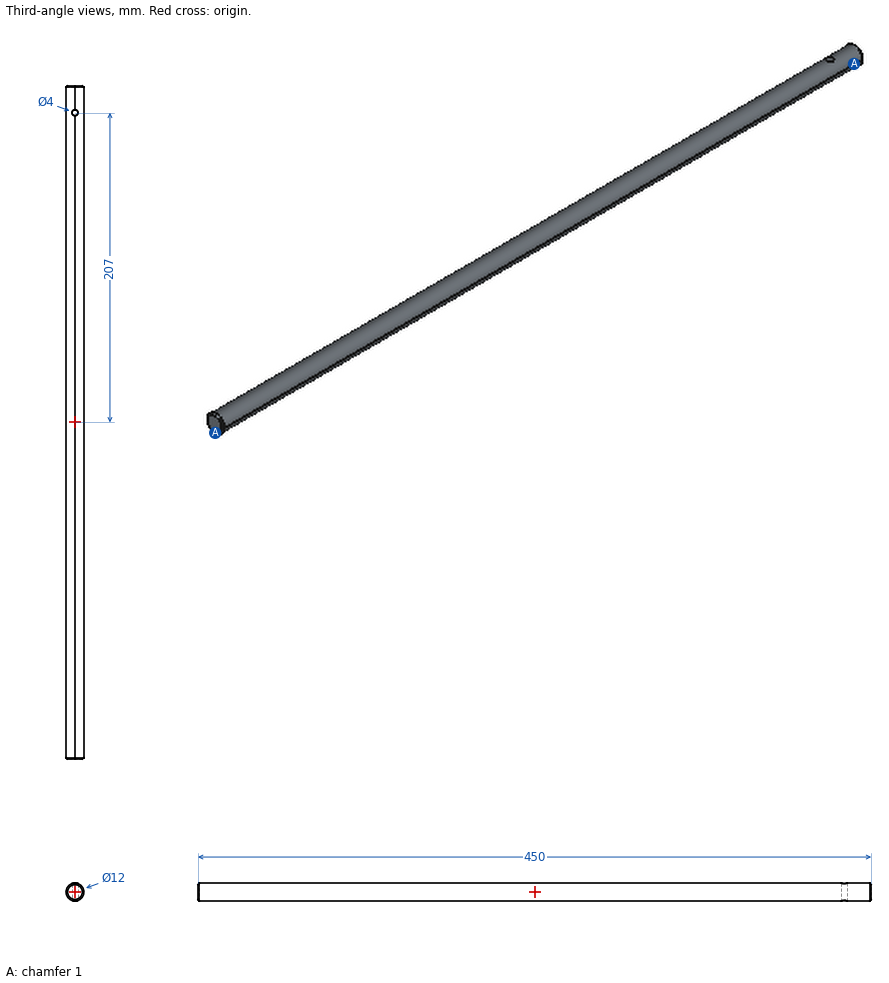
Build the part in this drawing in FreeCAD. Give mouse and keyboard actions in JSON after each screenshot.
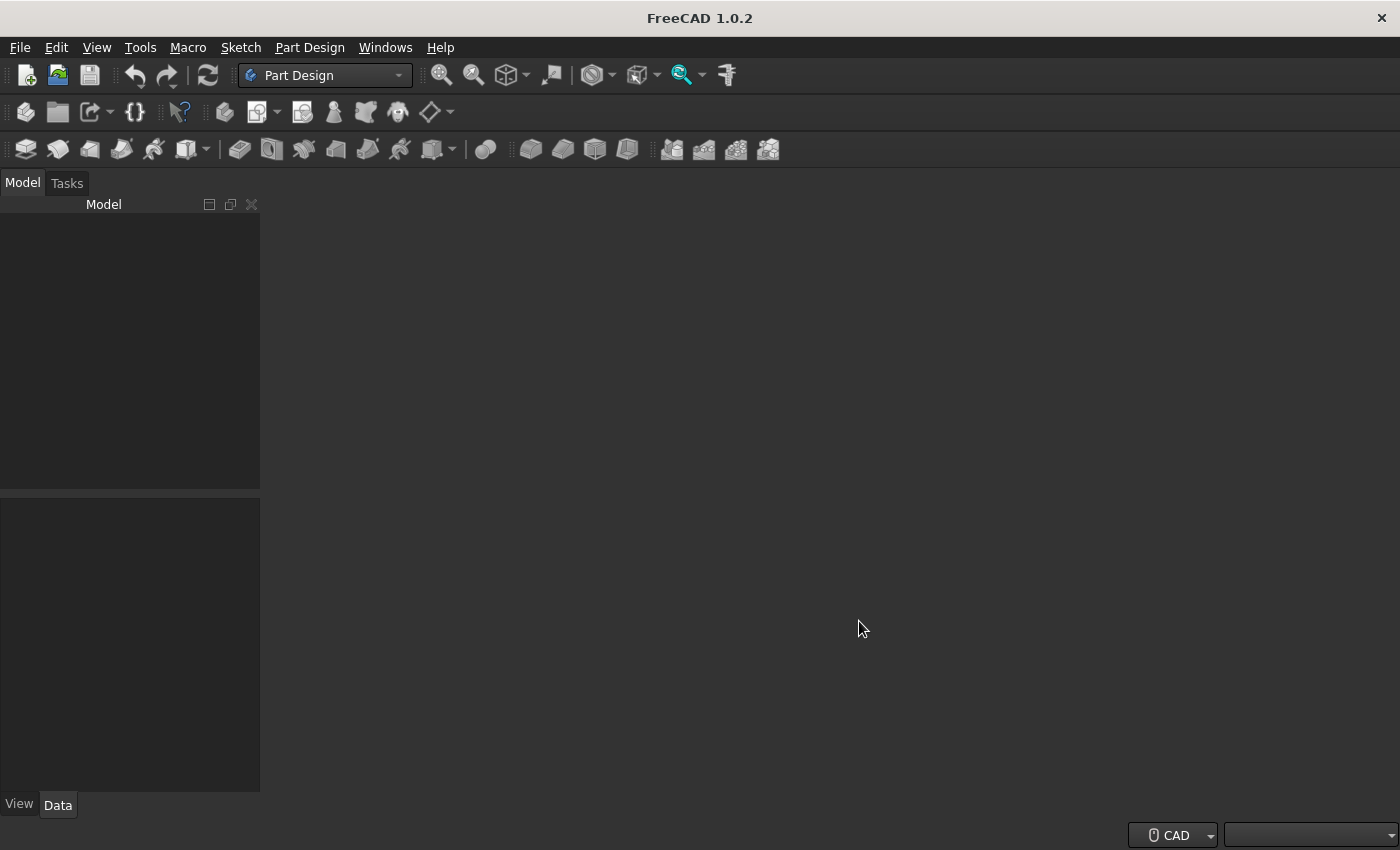
{"action": "key", "text": "ctrl+n"}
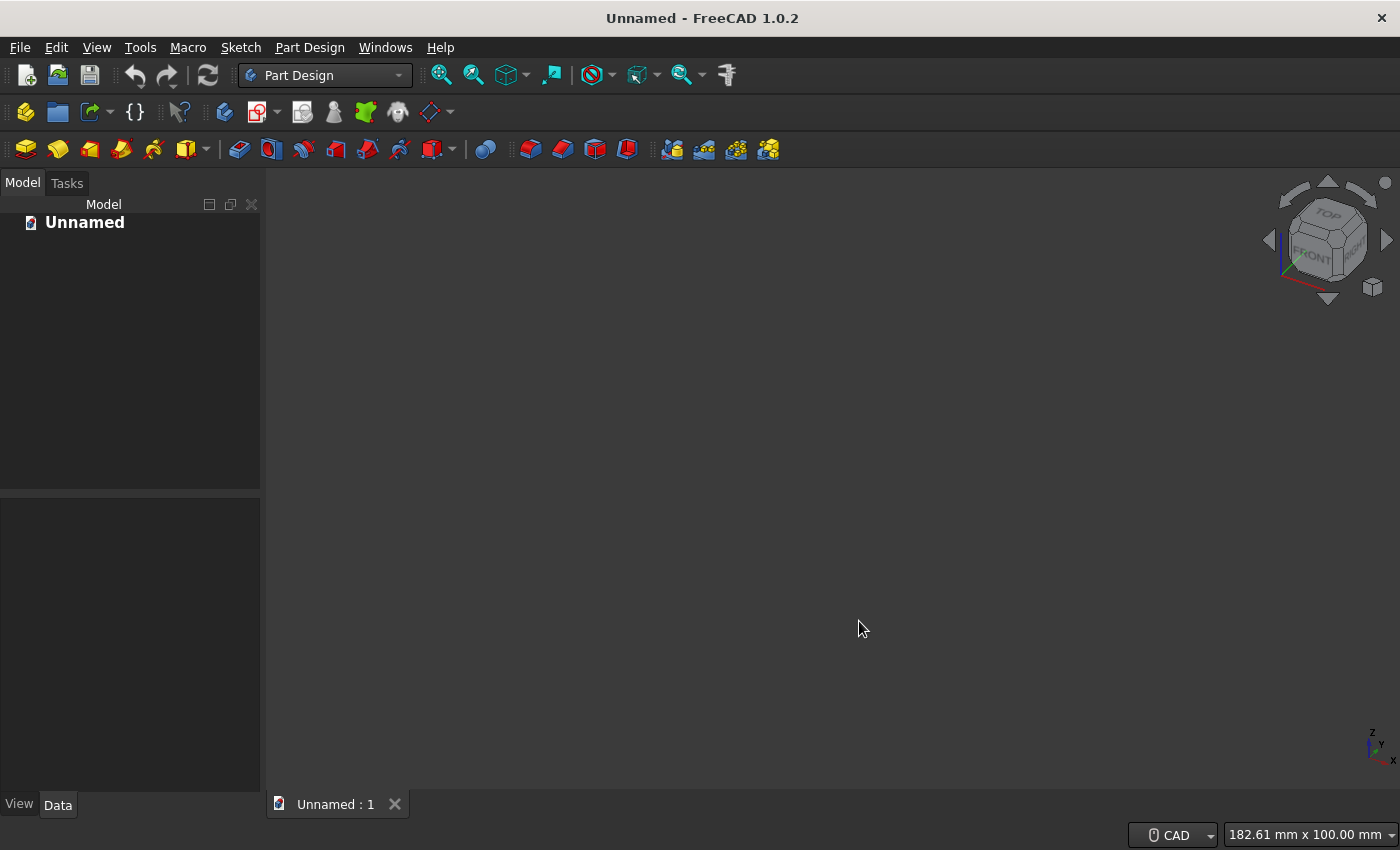
{"action": "left_click", "coordinate": [258, 112]}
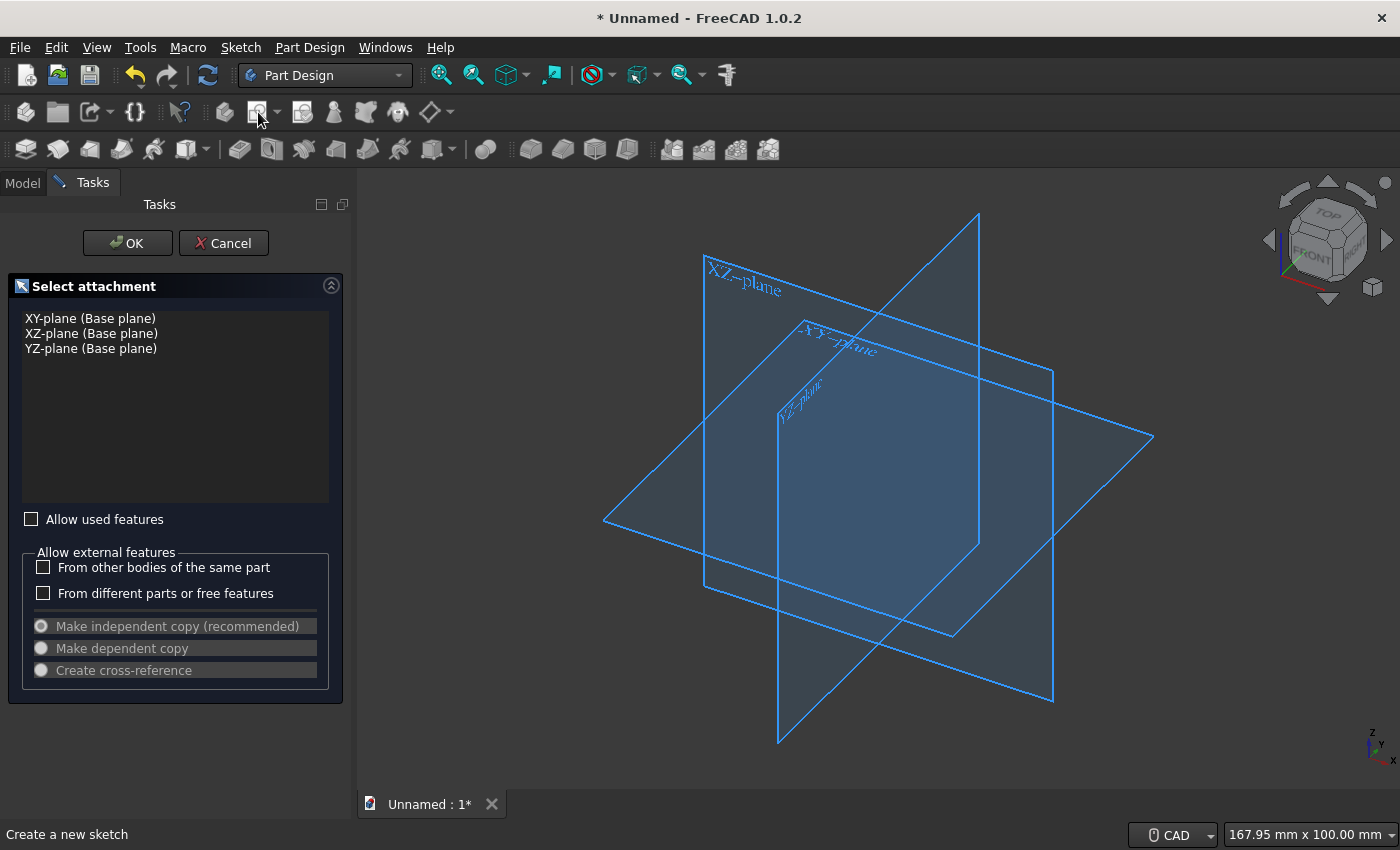
{"action": "left_click", "coordinate": [82, 334]}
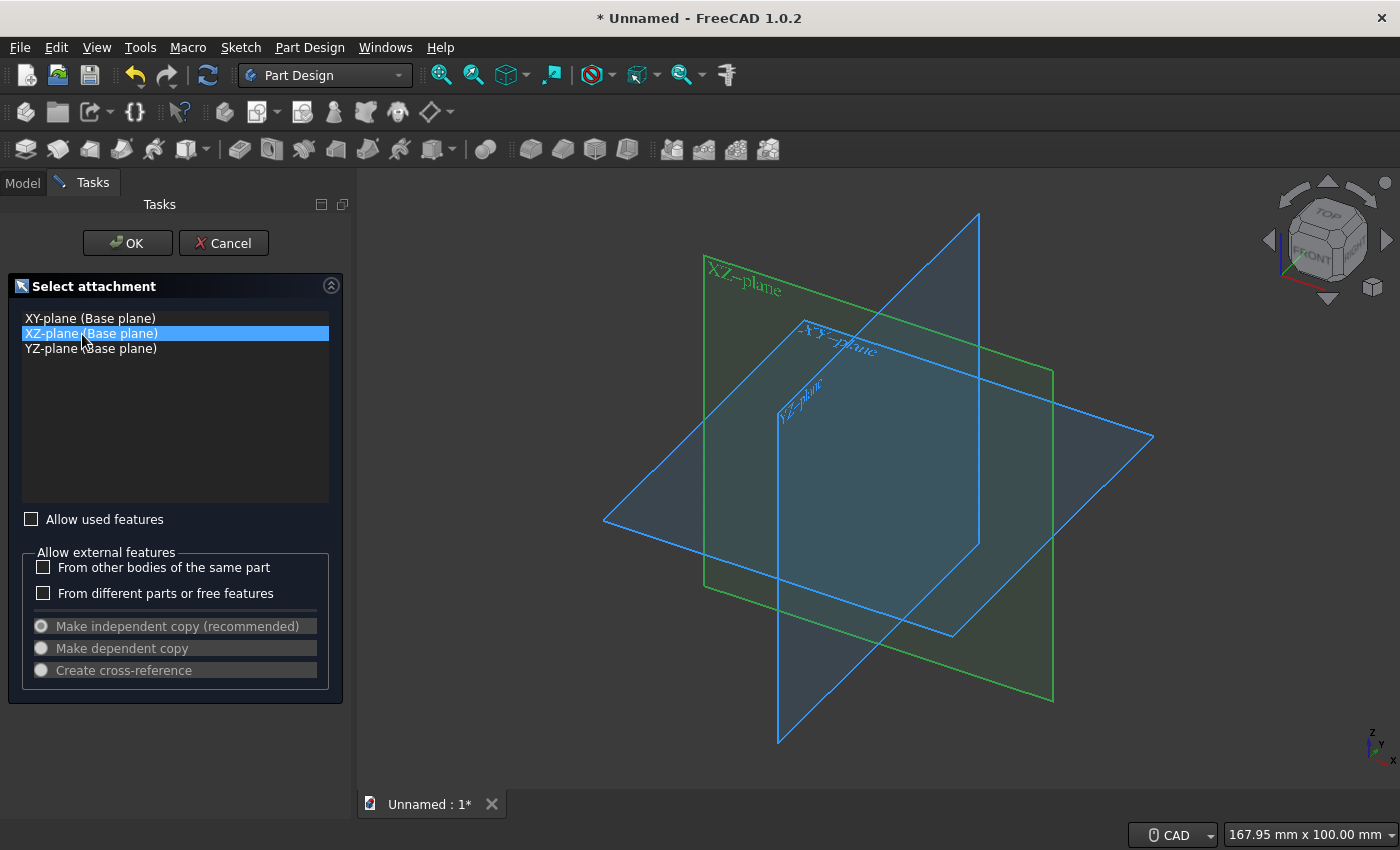
{"action": "left_click", "coordinate": [128, 243]}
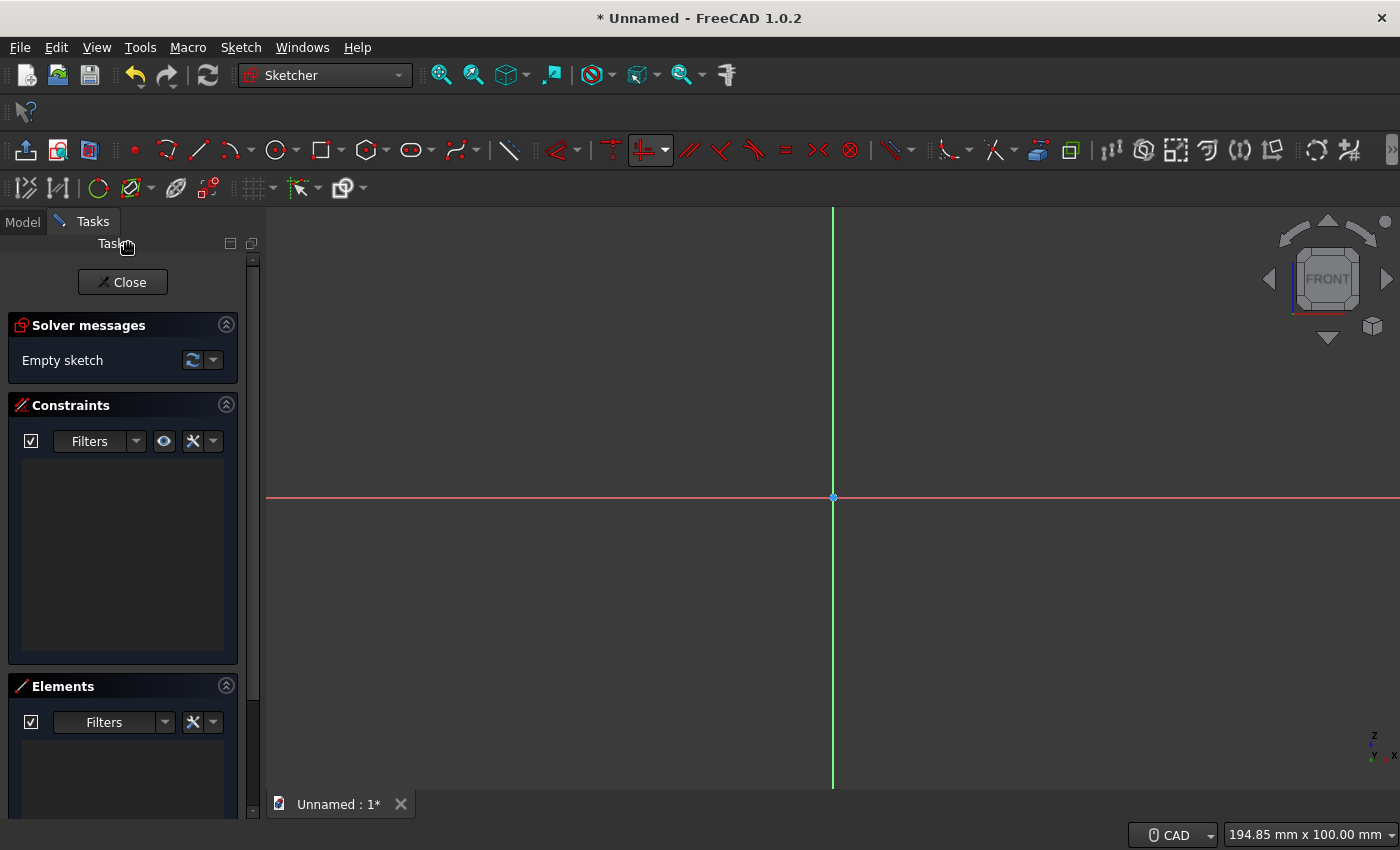
{"action": "scroll", "coordinate": [850, 498], "scroll_direction": "up", "scroll_amount": 8}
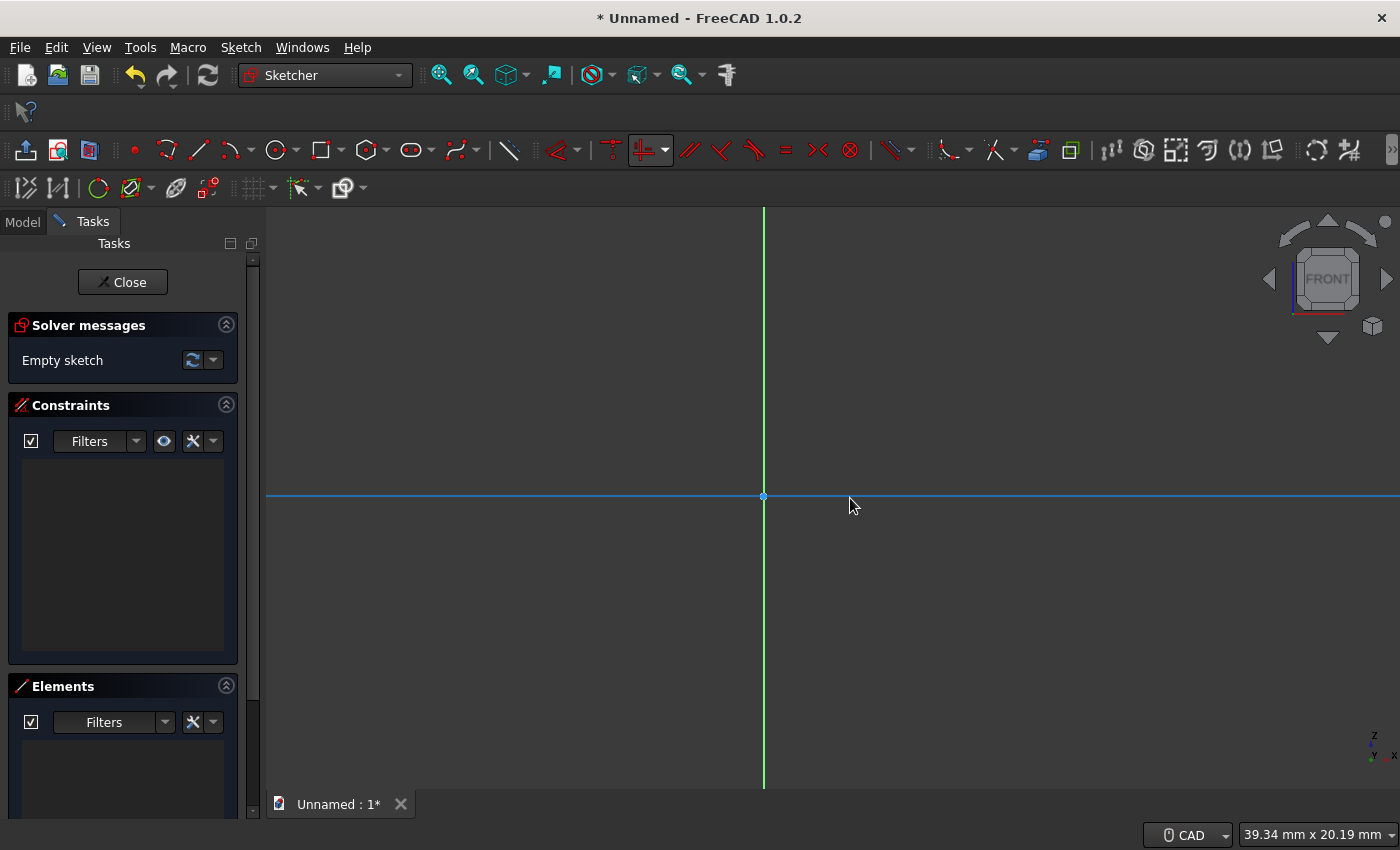
{"action": "key", "text": "g c"}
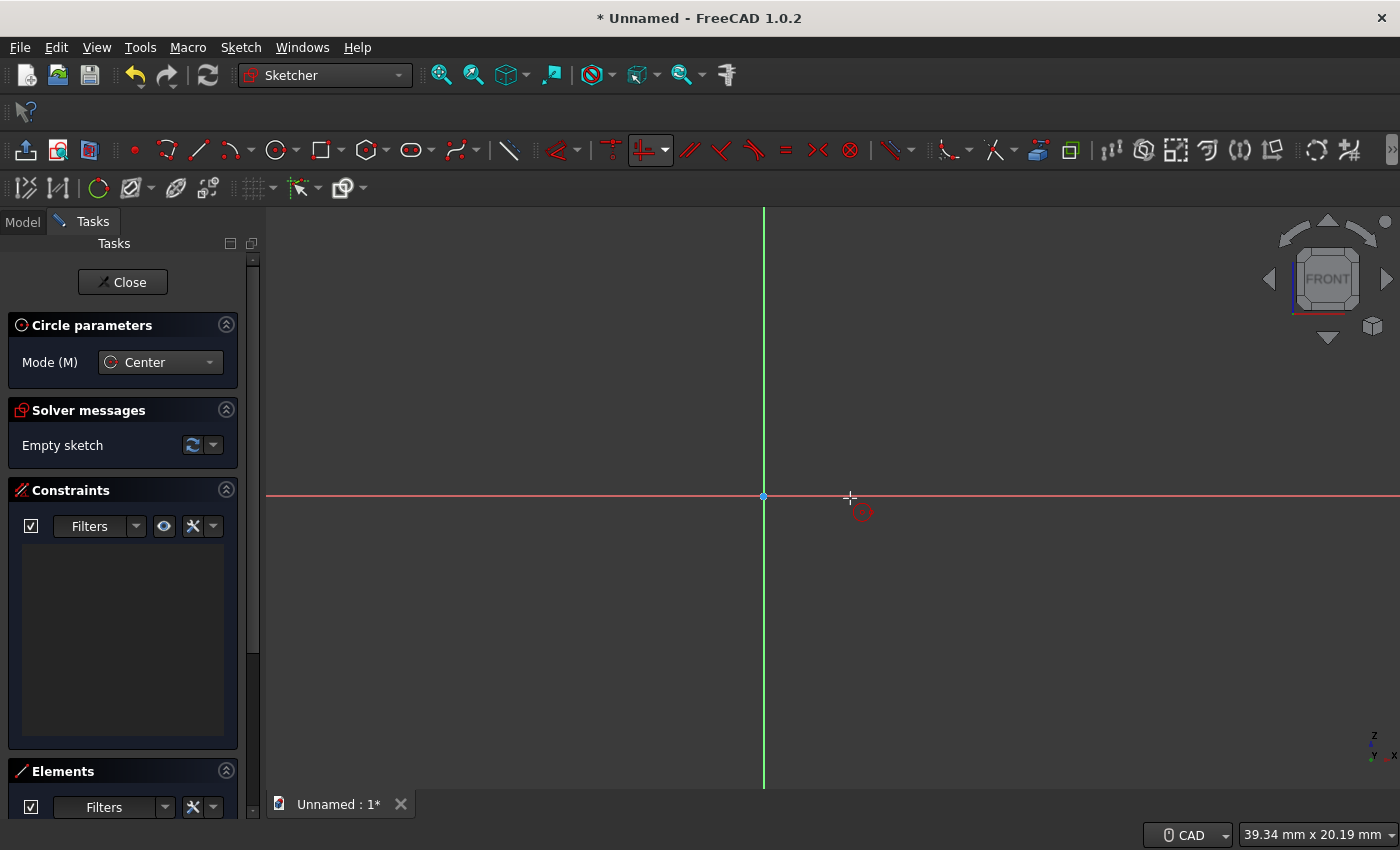
{"action": "left_click", "coordinate": [764, 496]}
{"action": "left_click", "coordinate": [886, 374]}
{"action": "key", "text": "Escape"}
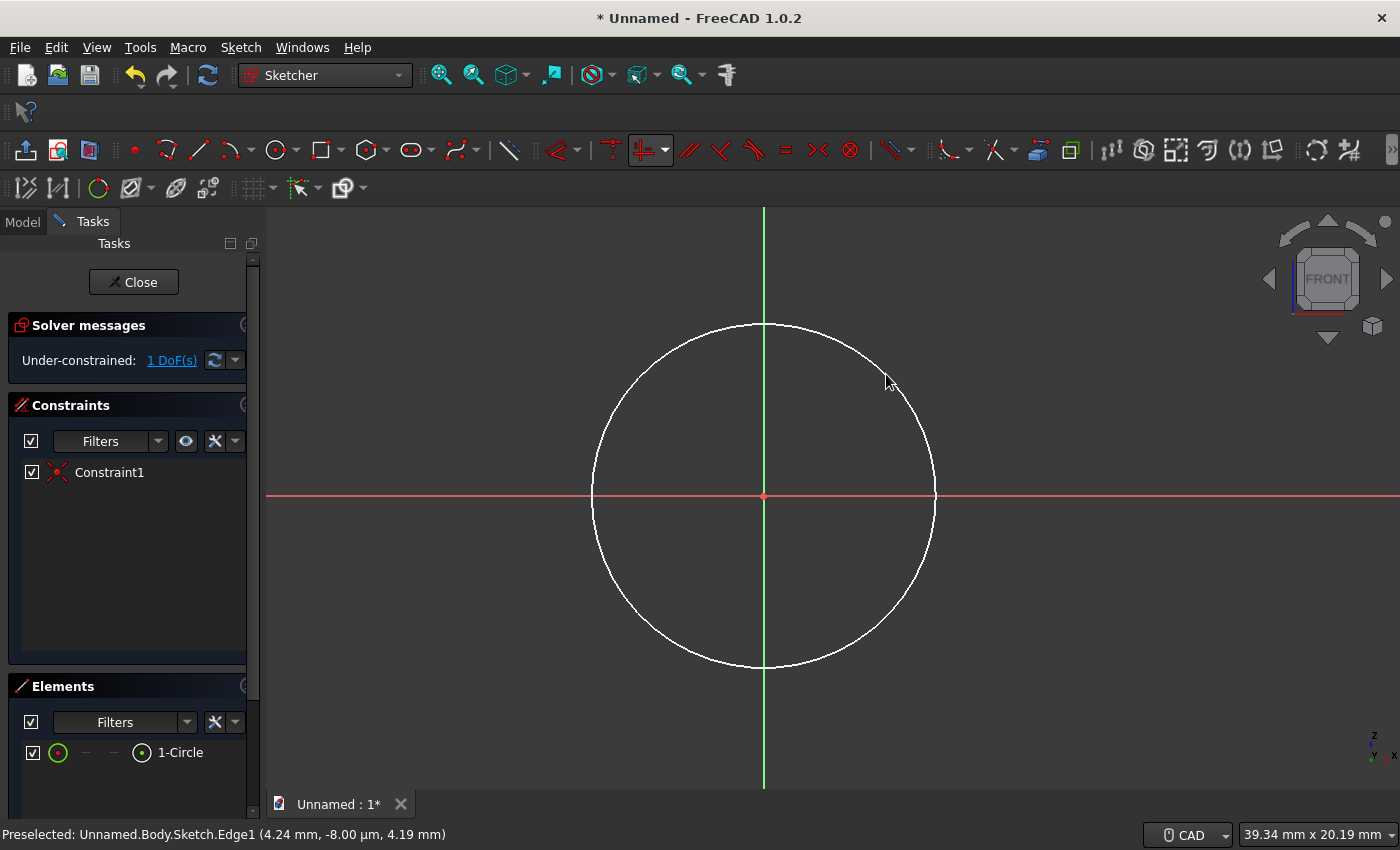
{"action": "key", "text": "d"}